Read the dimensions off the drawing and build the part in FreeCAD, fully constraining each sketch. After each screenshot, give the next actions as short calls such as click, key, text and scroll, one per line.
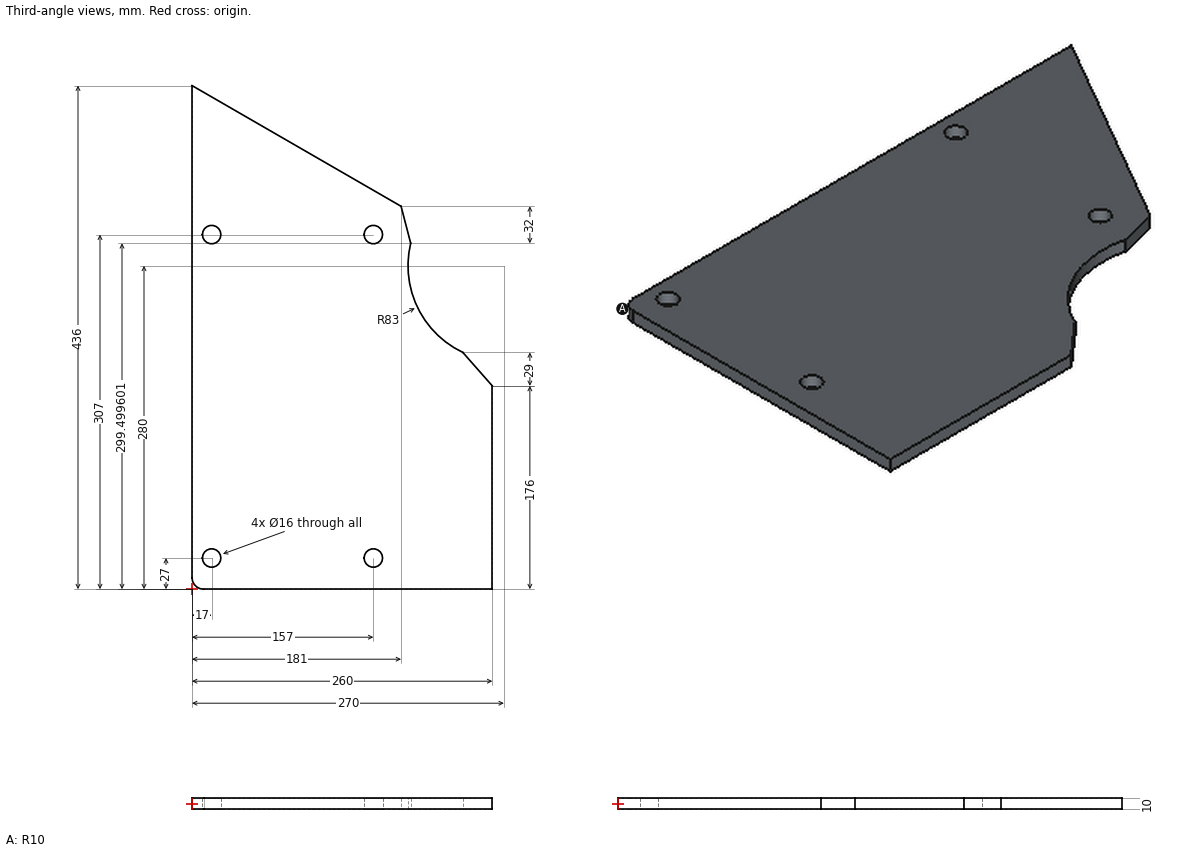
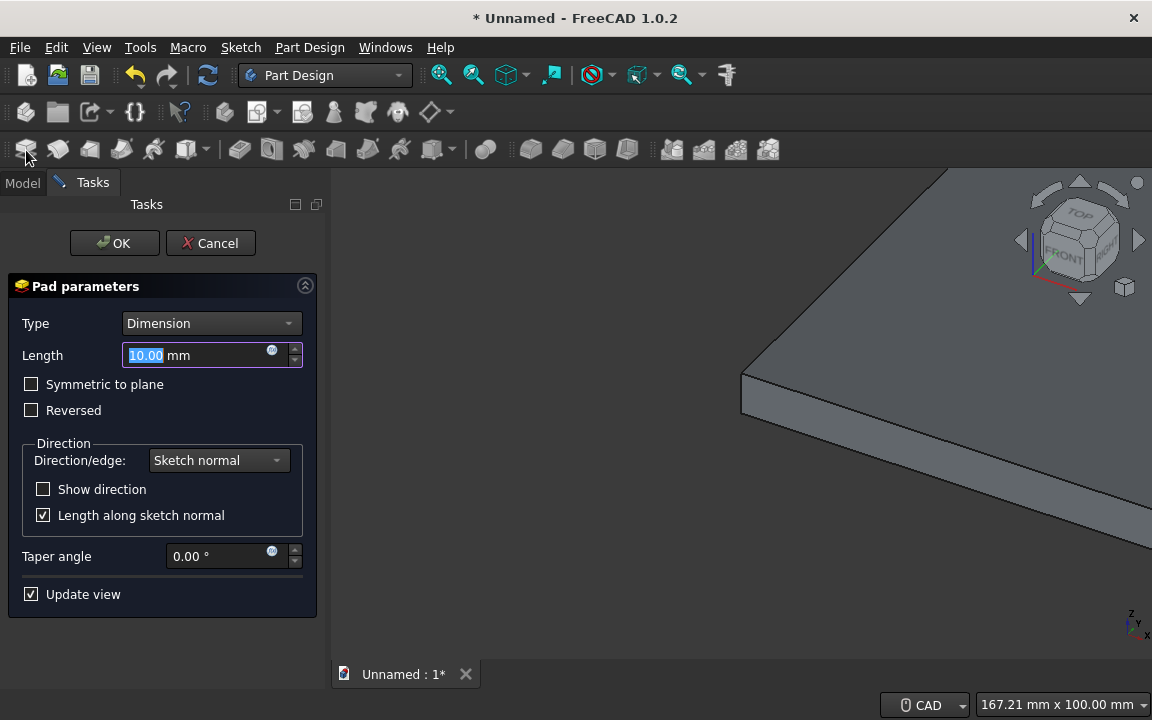
text(10)
key(Tab)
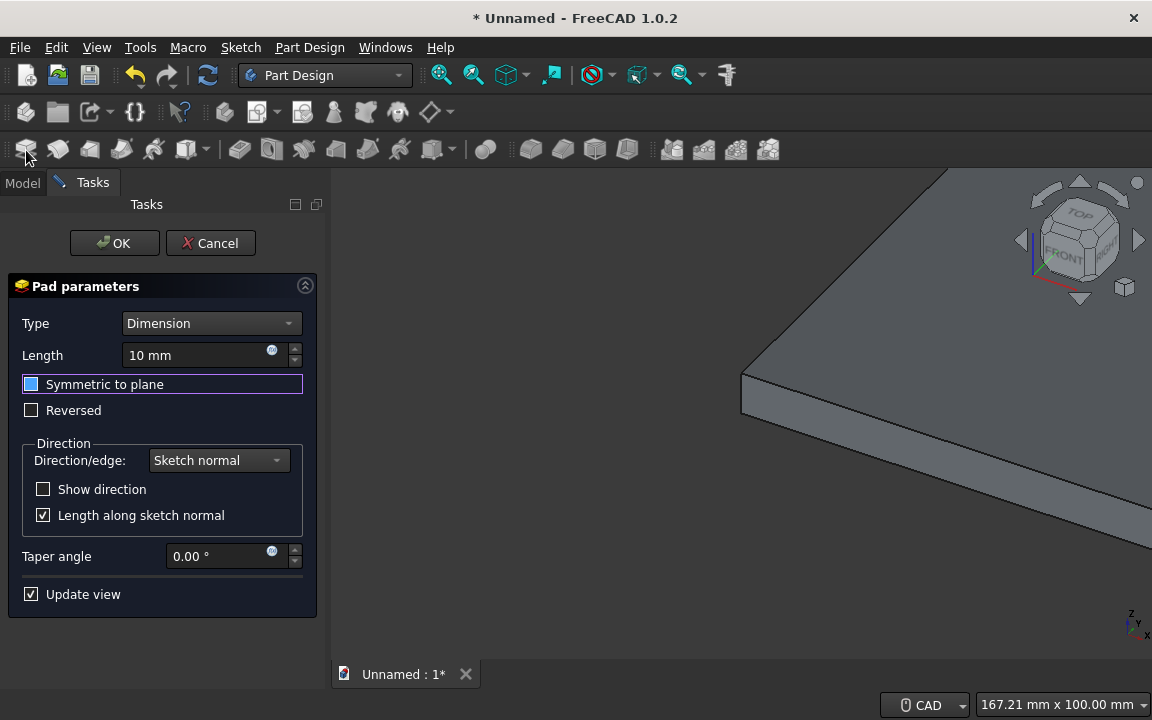
click(30, 384)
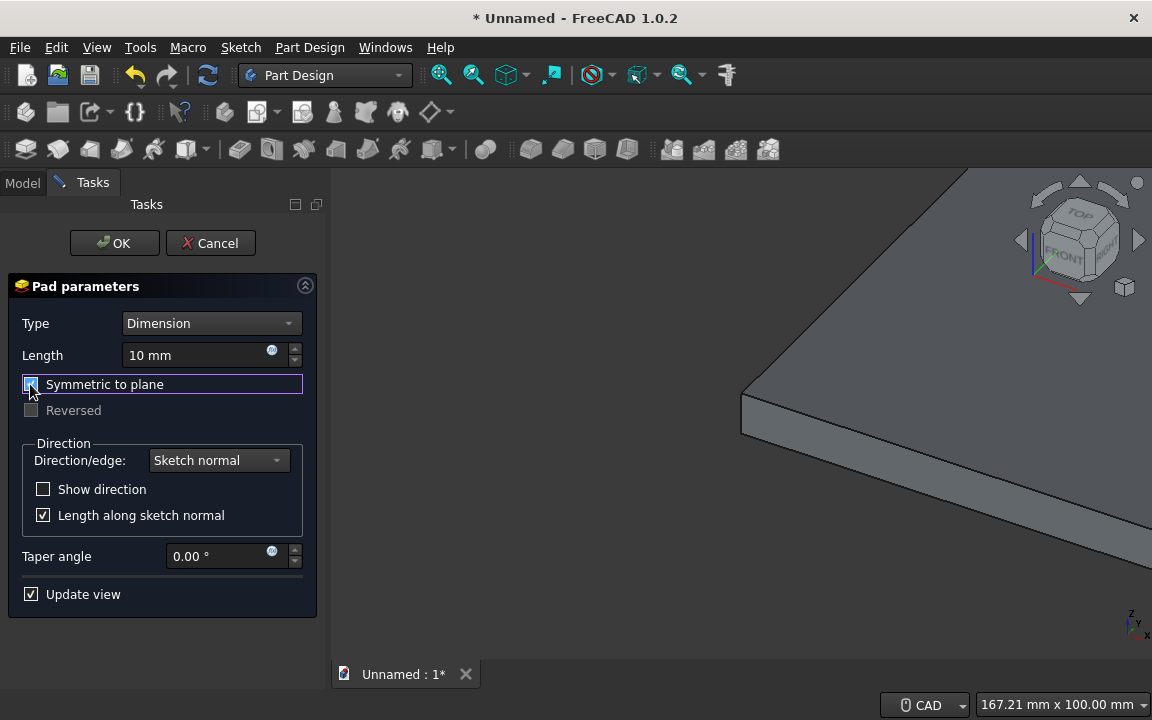
click(115, 243)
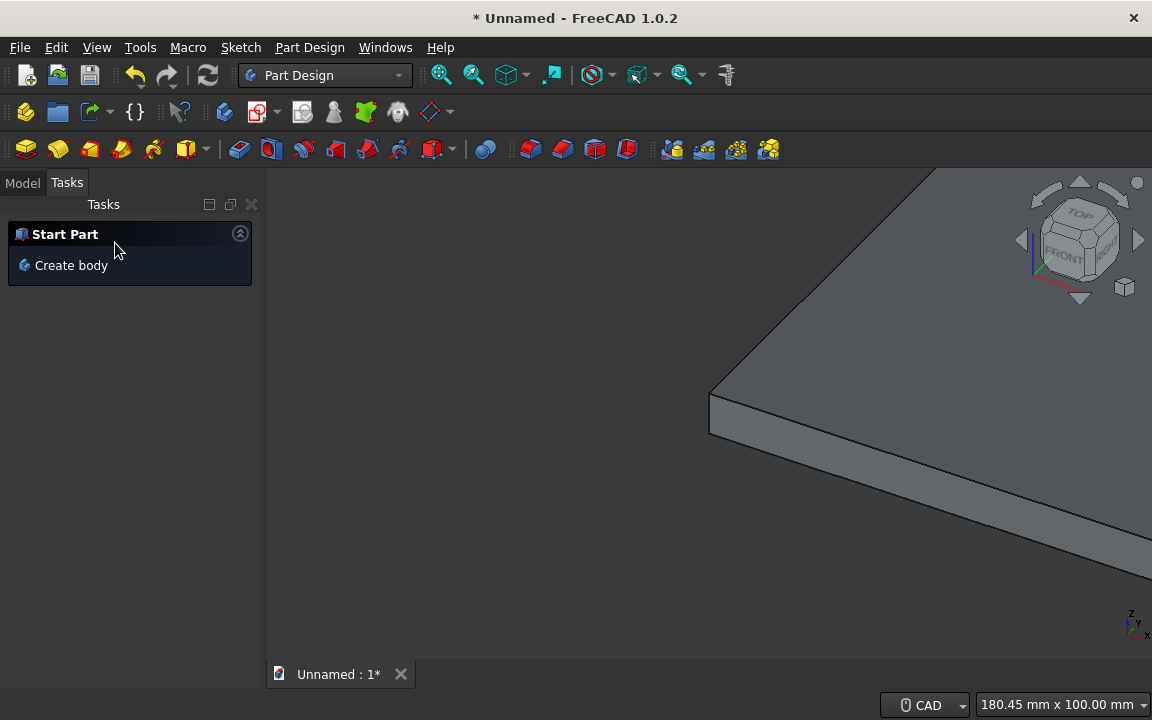
key(v)
key(f)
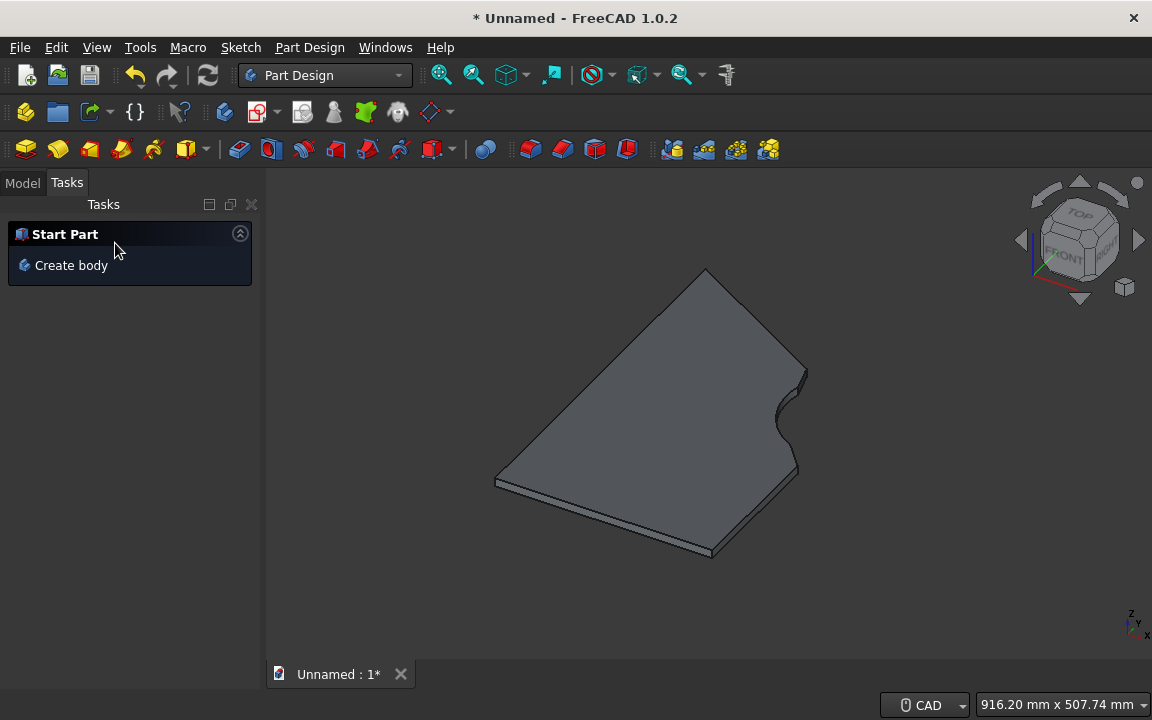
click(679, 438)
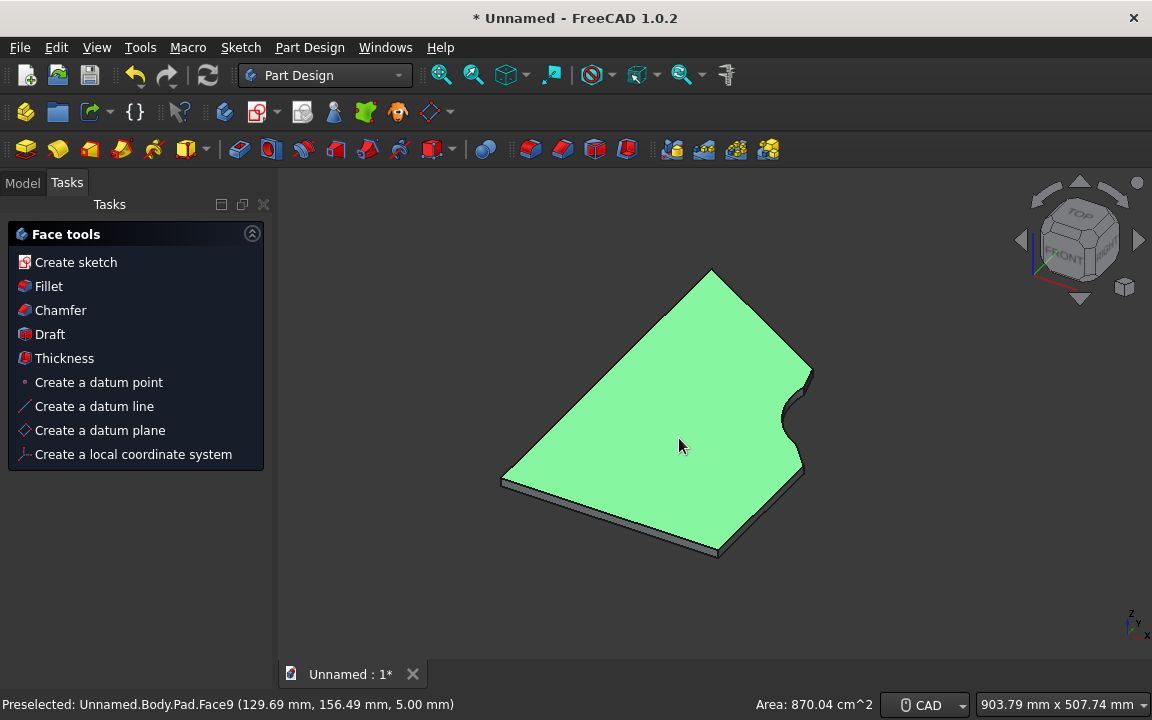
click(258, 112)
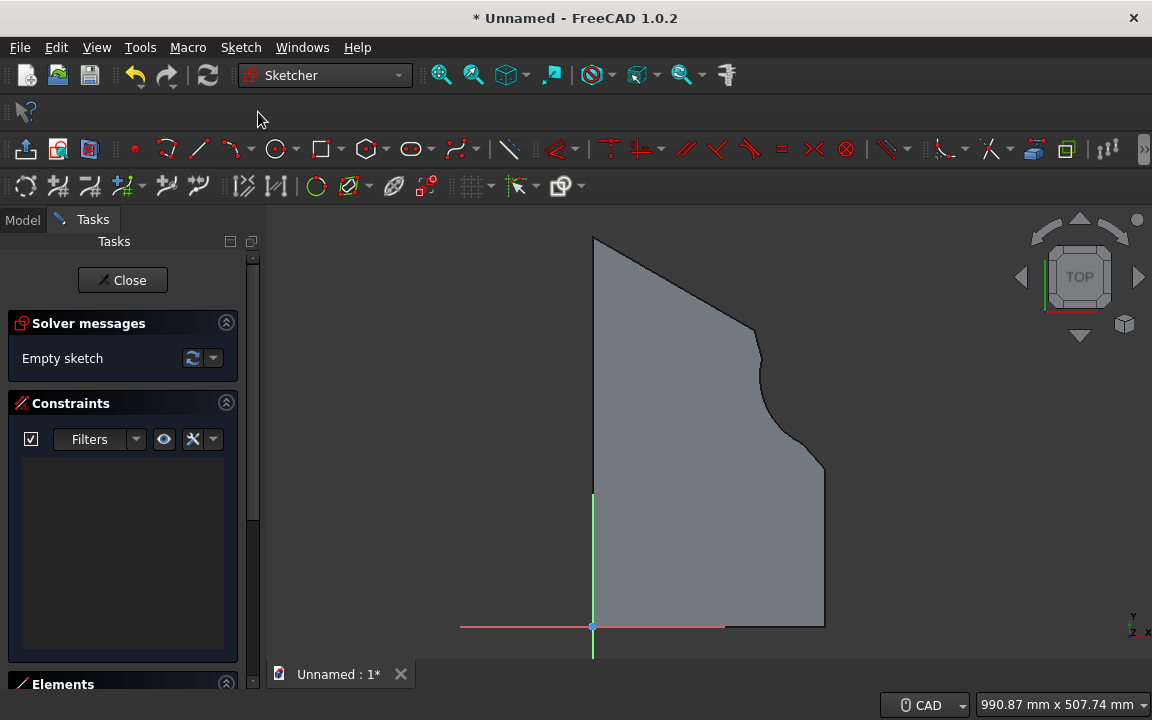
scroll(523, 233, down, 1)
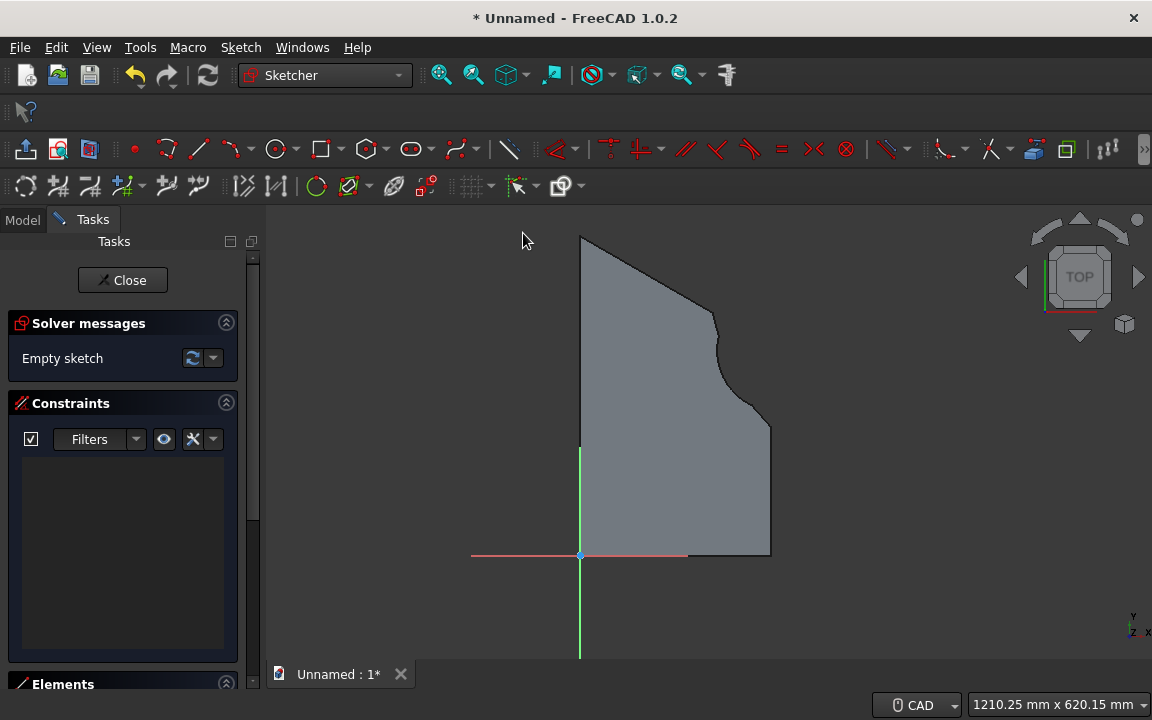
key(g)
key(c)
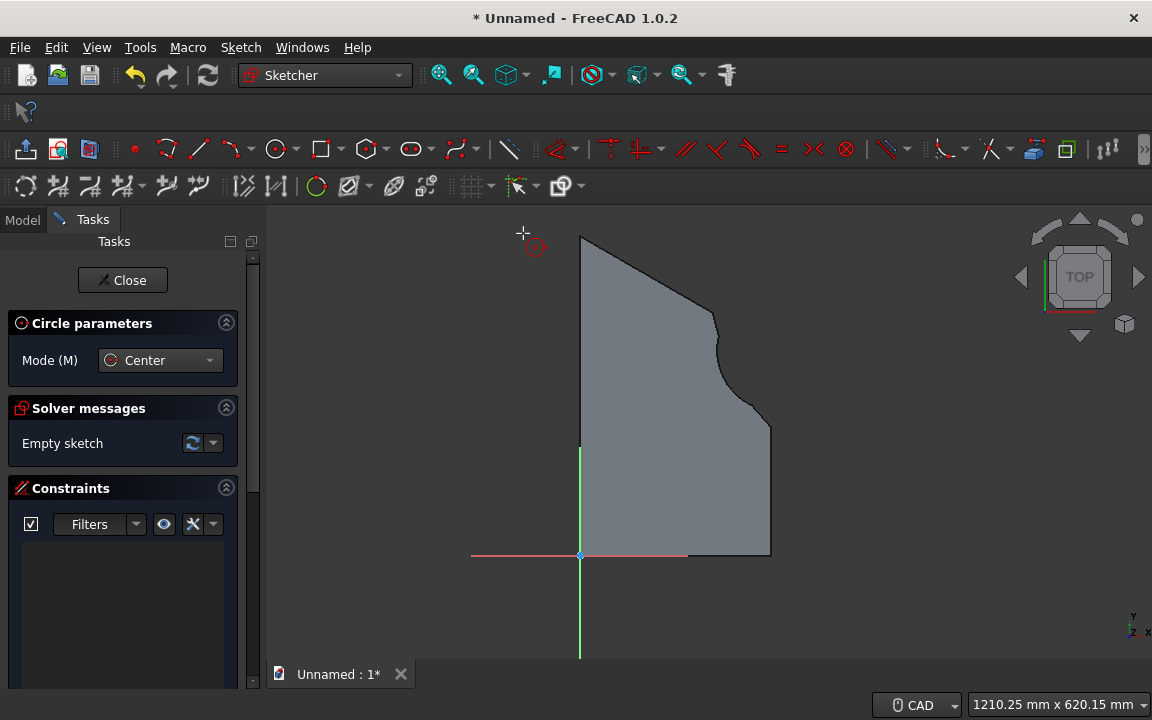
scroll(593, 536, up, 7)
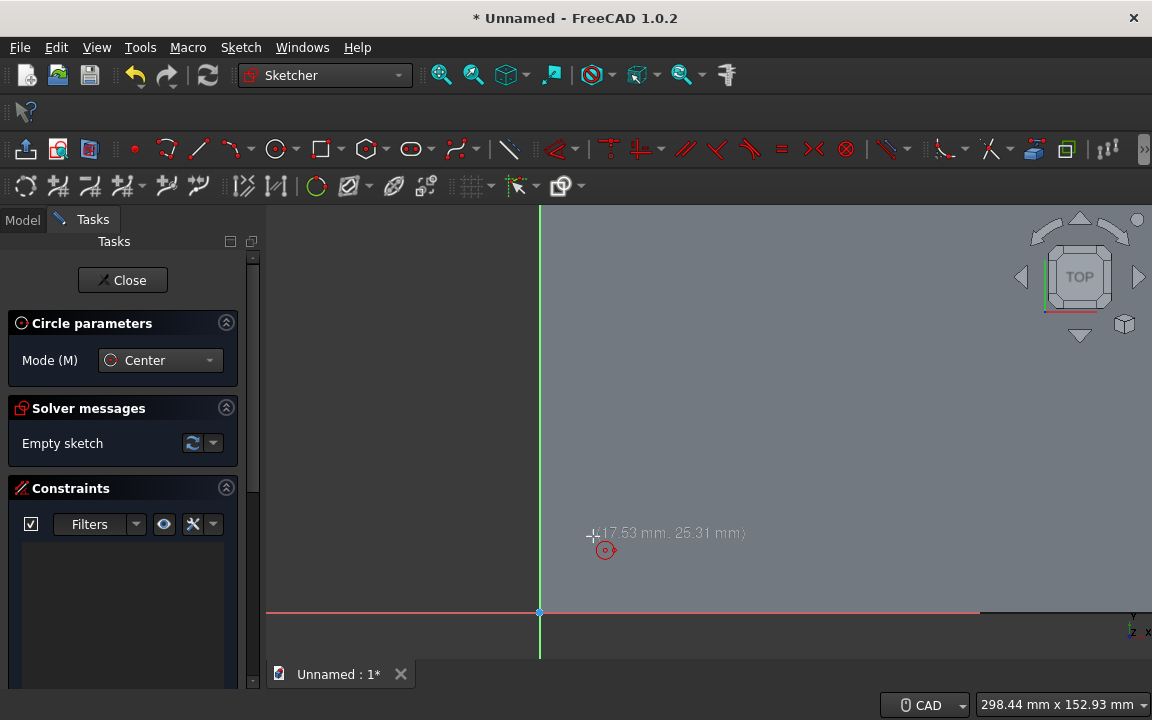
scroll(578, 556, down, 6)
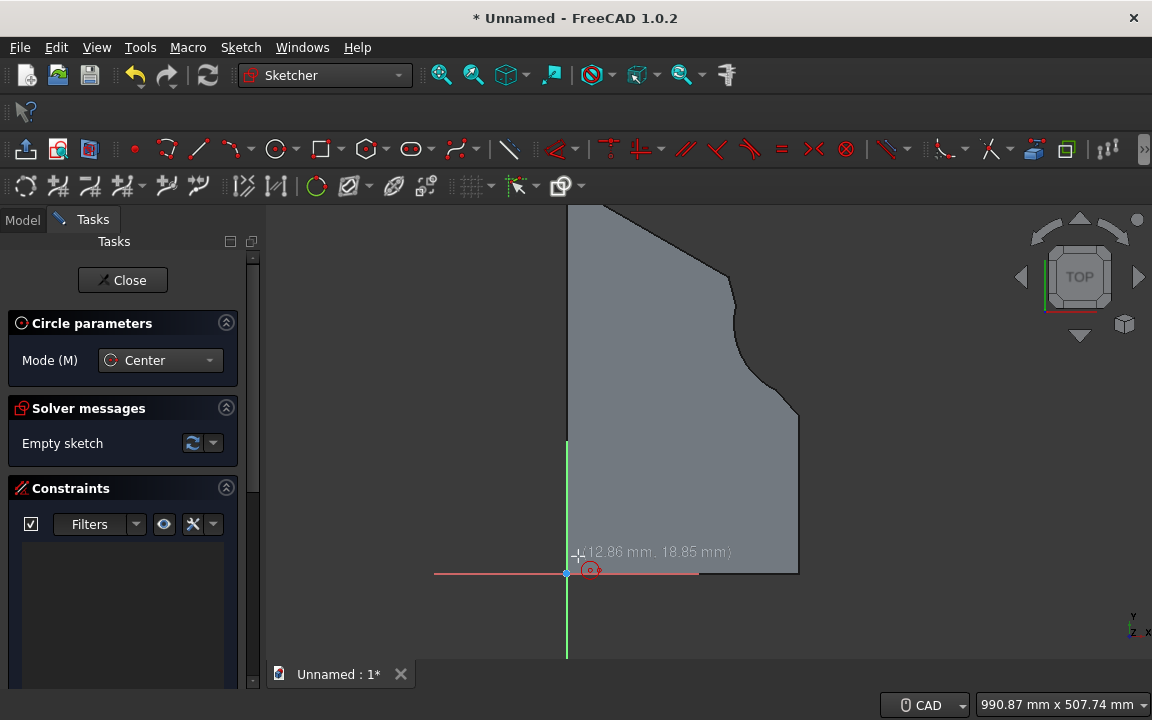
click(582, 550)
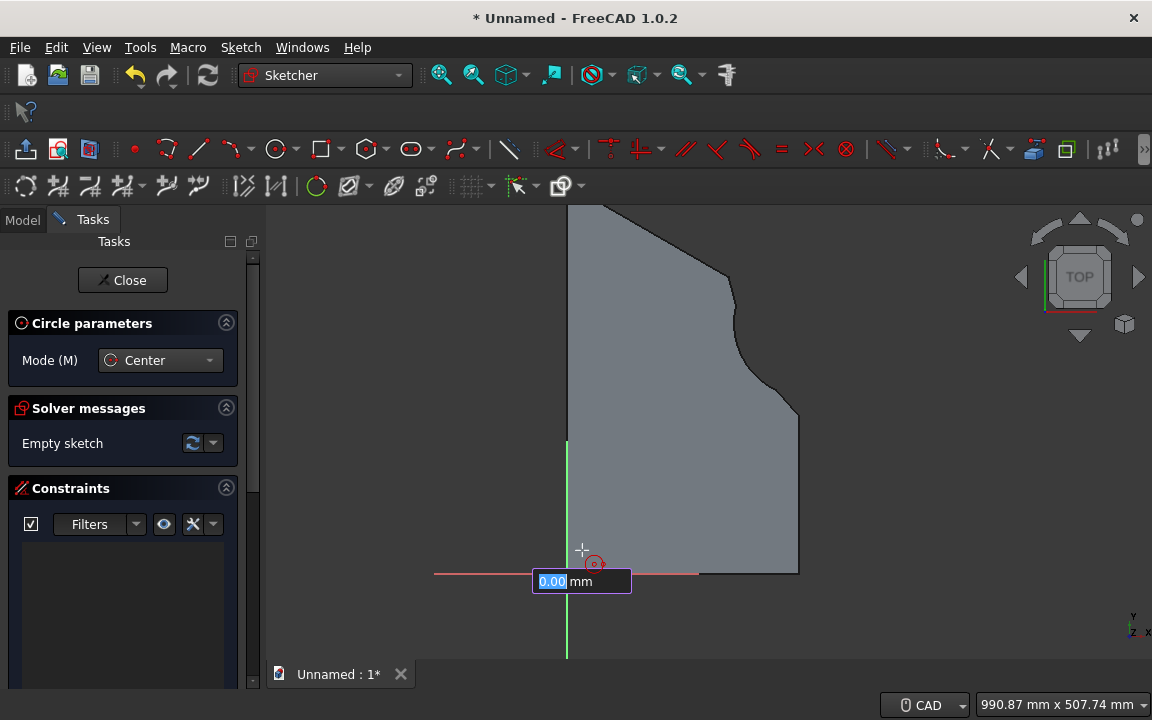
scroll(587, 545, up, 4)